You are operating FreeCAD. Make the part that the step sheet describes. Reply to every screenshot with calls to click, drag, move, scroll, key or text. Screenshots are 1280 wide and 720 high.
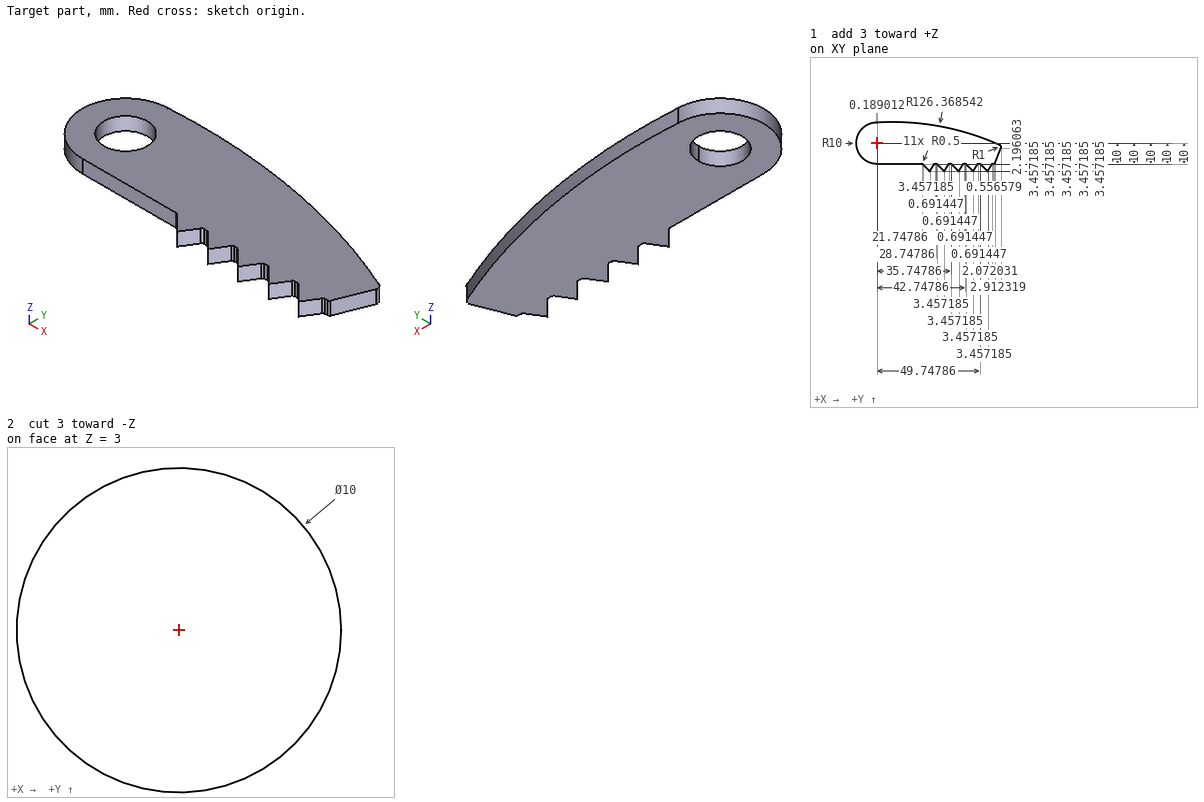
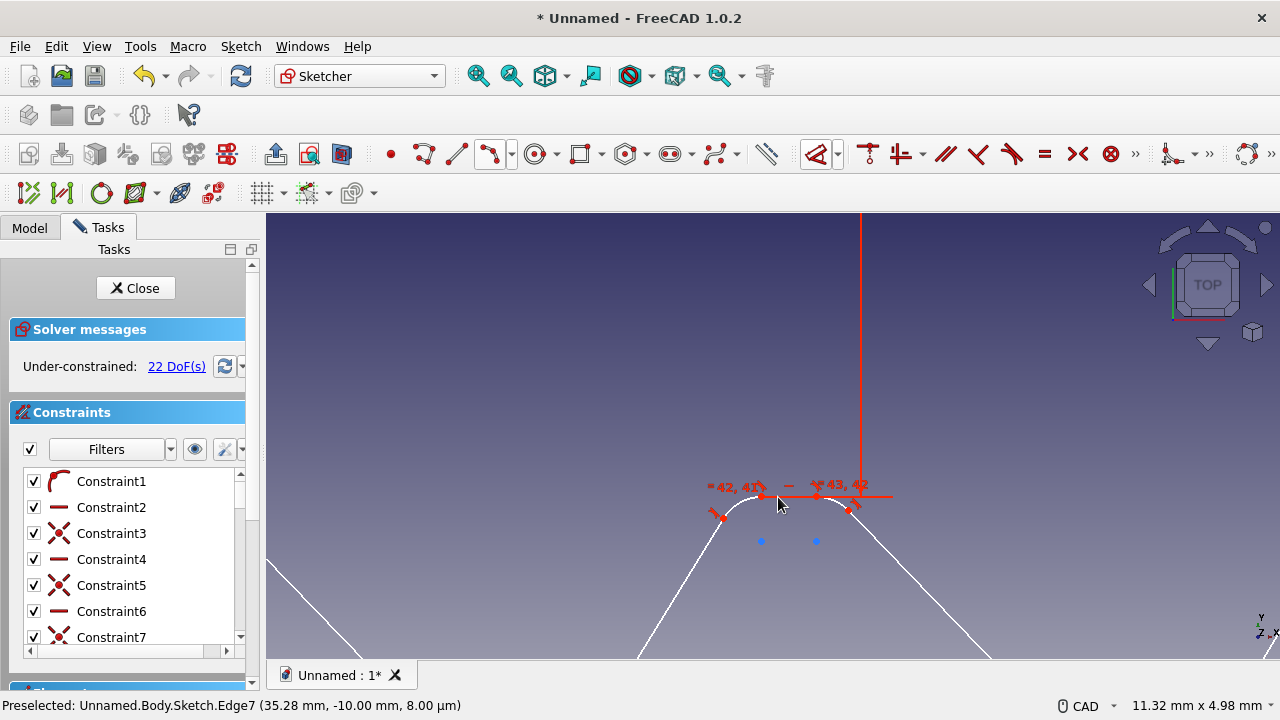
click(838, 154)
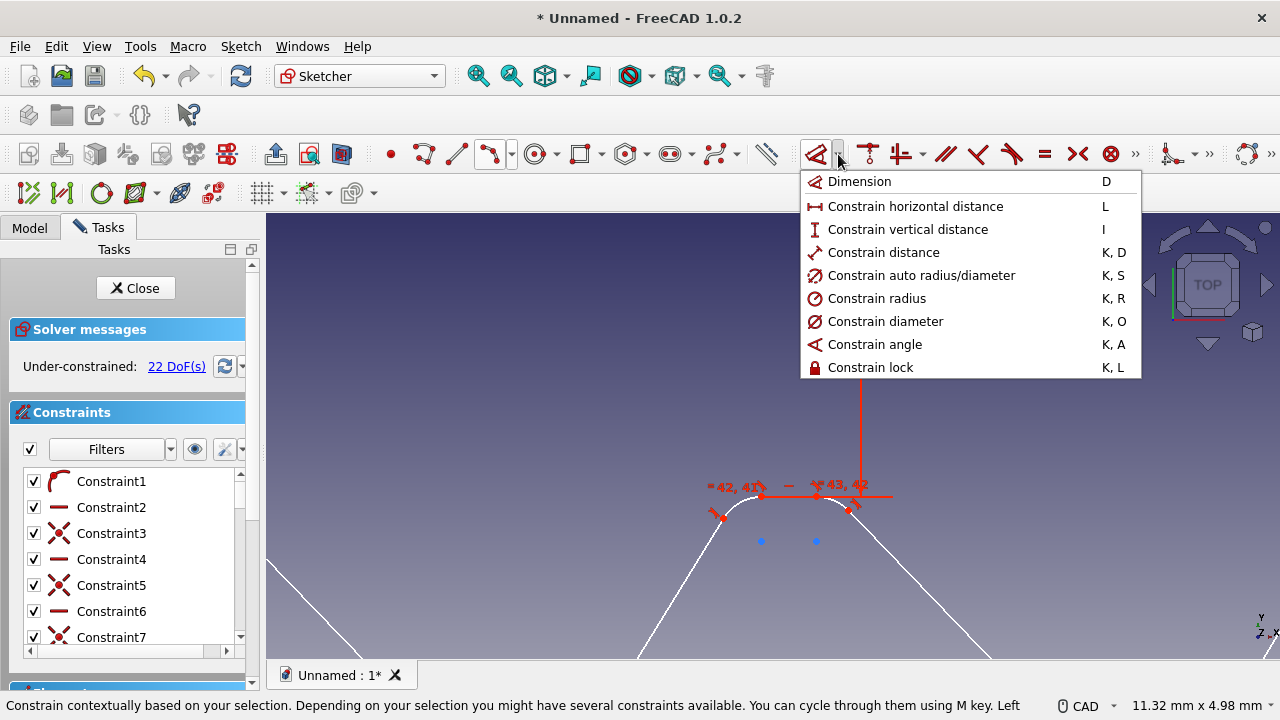
click(971, 206)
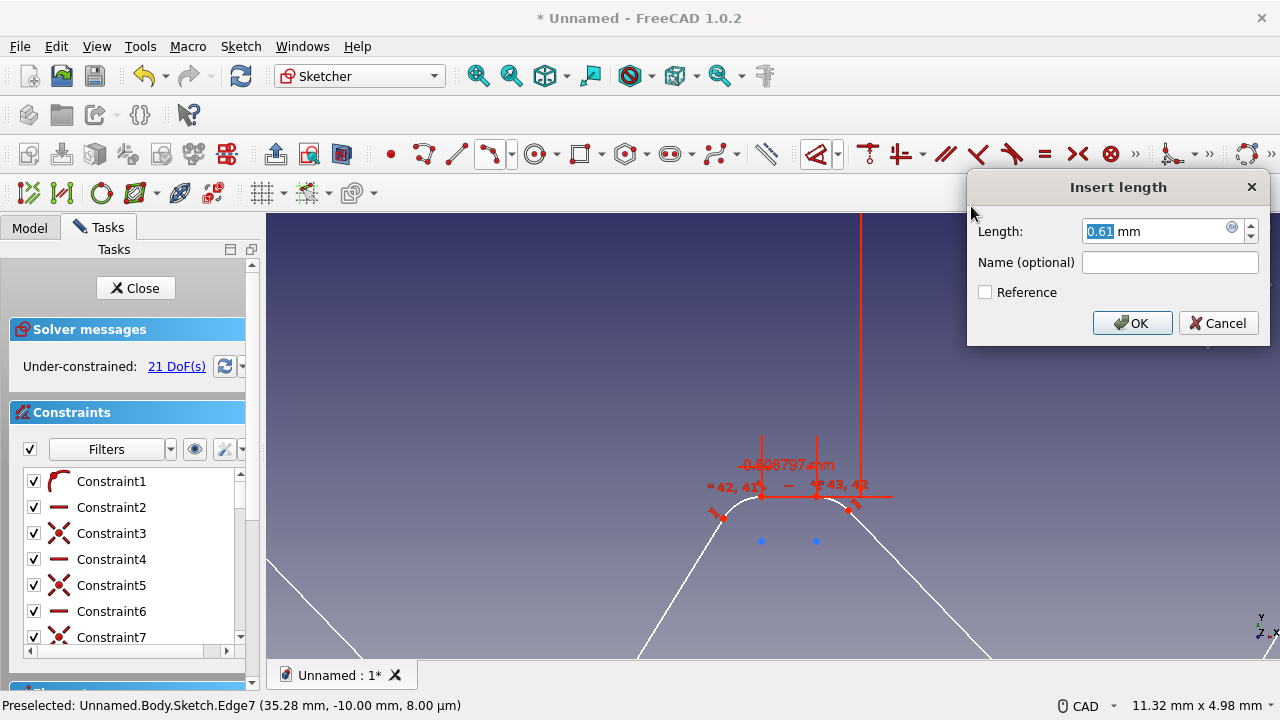
text(0.691447)
key(Return)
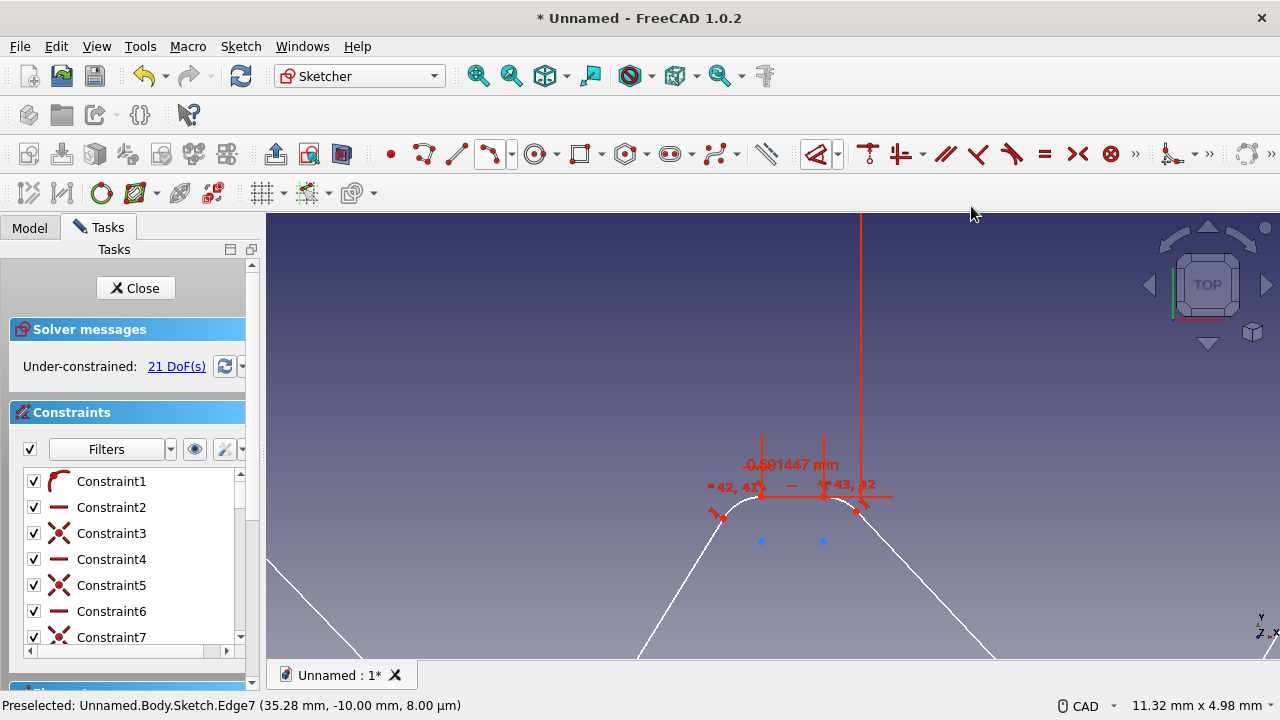
scroll(789, 503, down, 12)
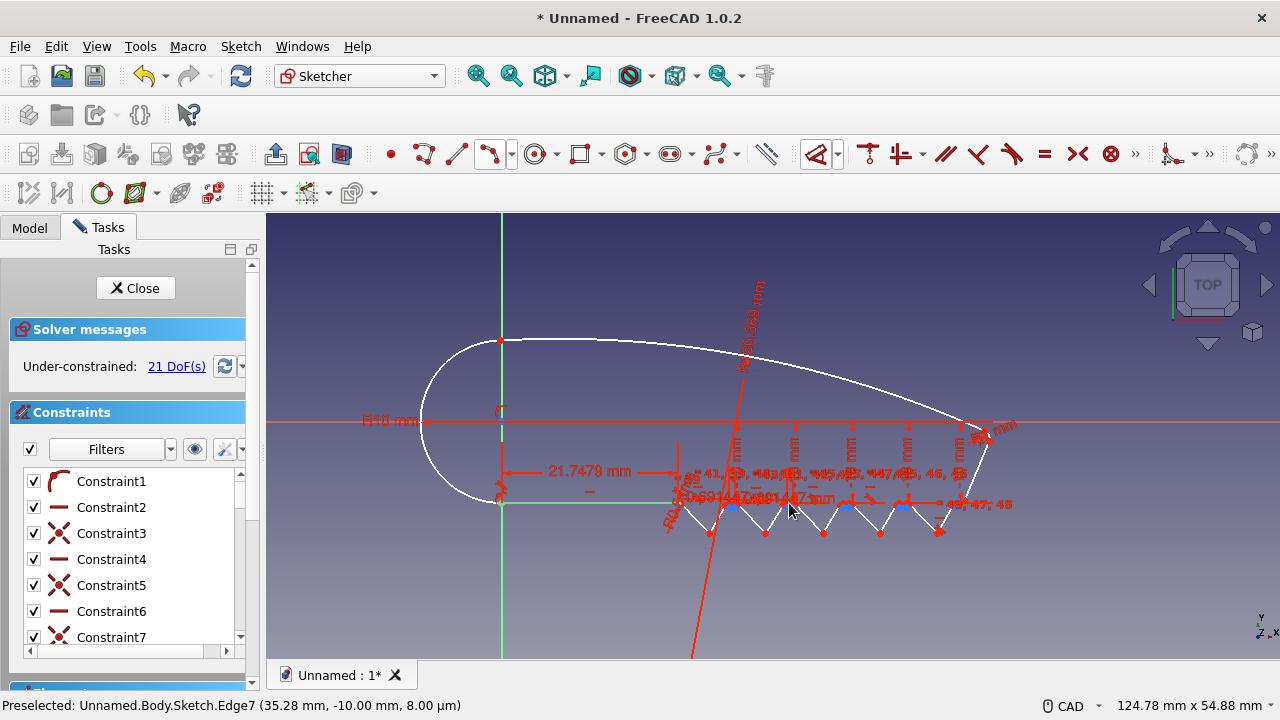
scroll(845, 503, up, 11)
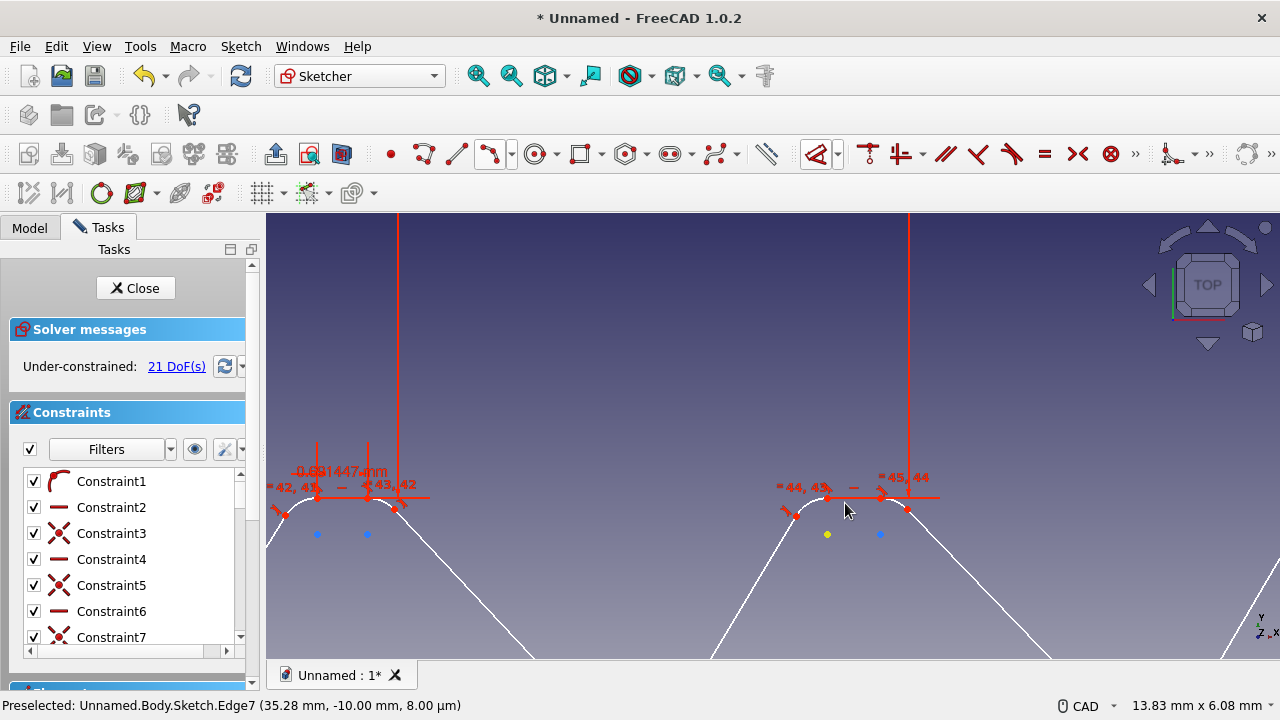
click(844, 498)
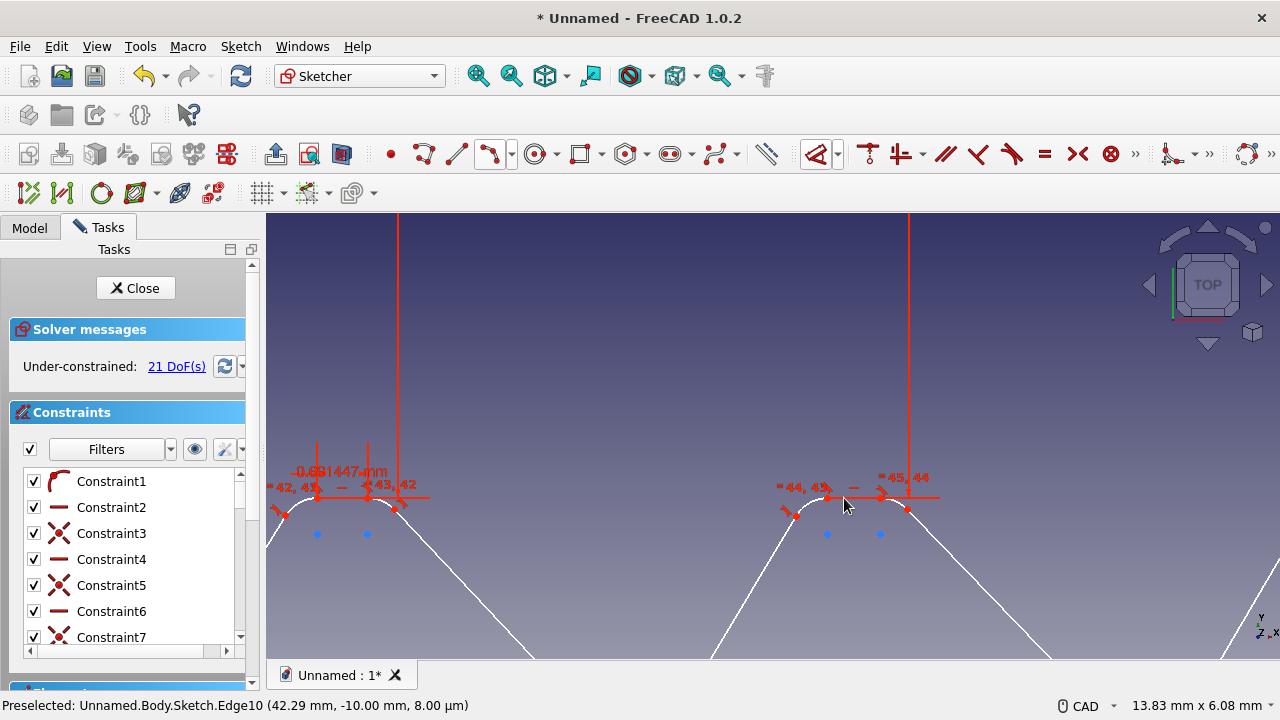
click(838, 154)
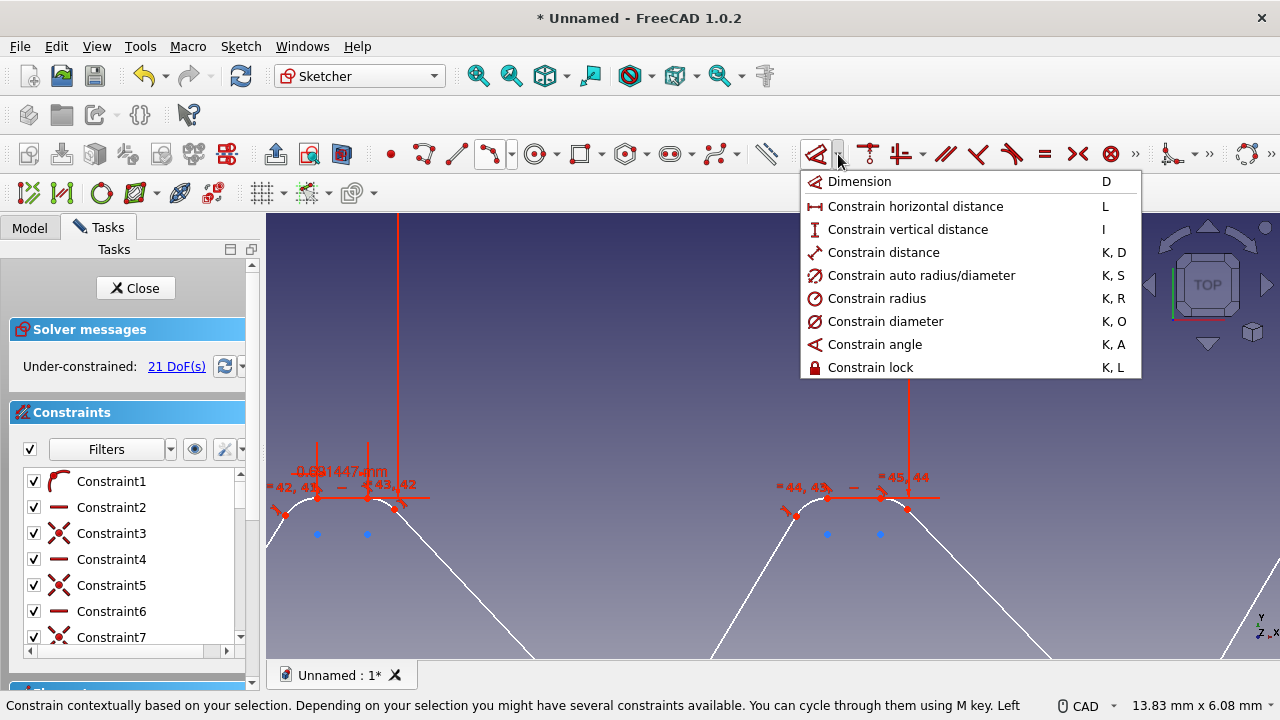
click(971, 206)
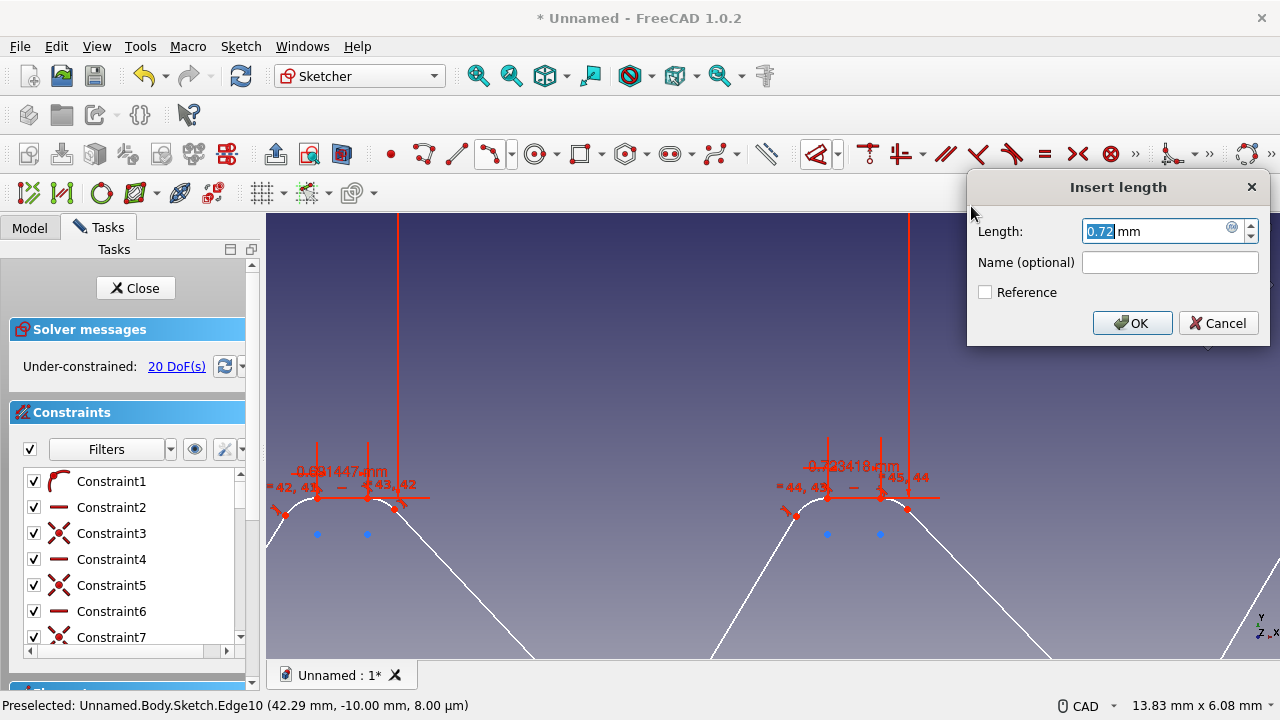
text(0.691447)
key(Return)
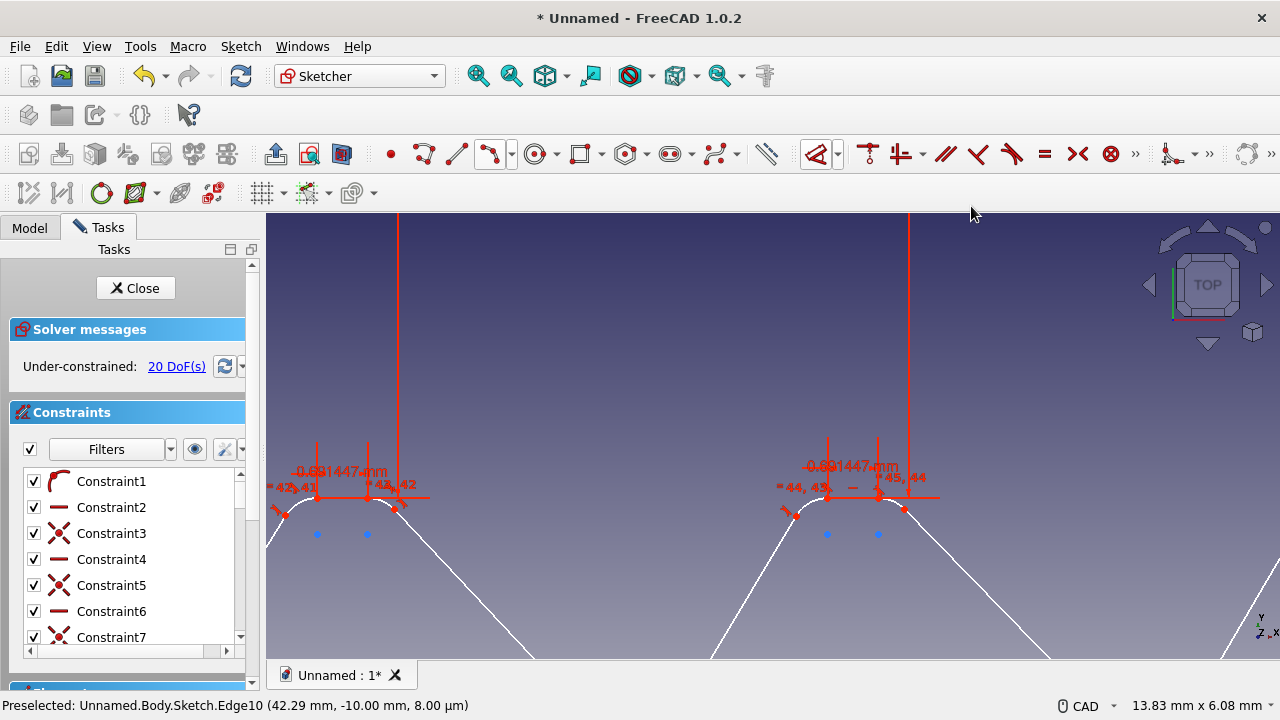
scroll(845, 503, down, 11)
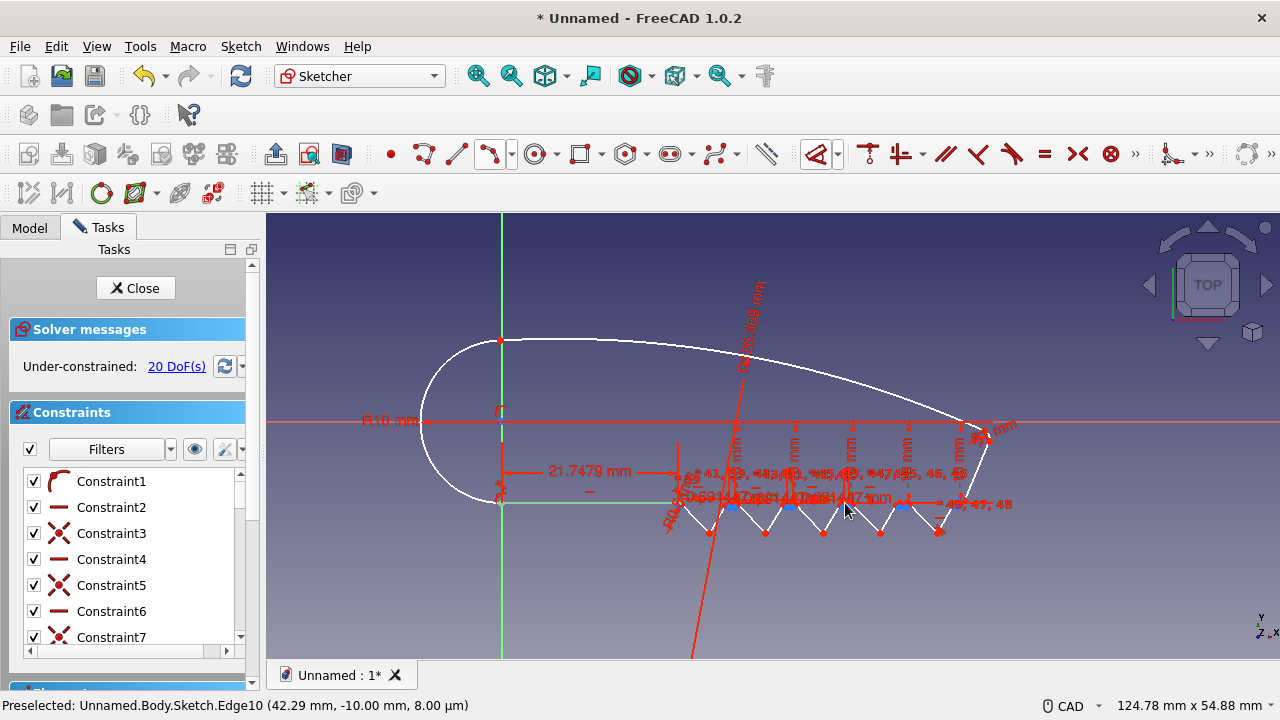
scroll(902, 503, up, 10)